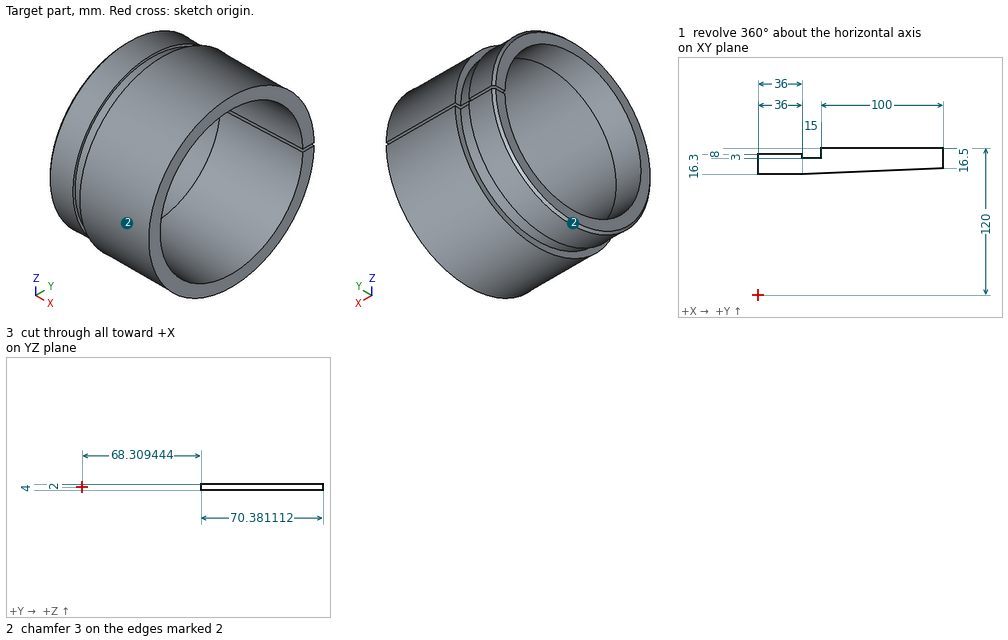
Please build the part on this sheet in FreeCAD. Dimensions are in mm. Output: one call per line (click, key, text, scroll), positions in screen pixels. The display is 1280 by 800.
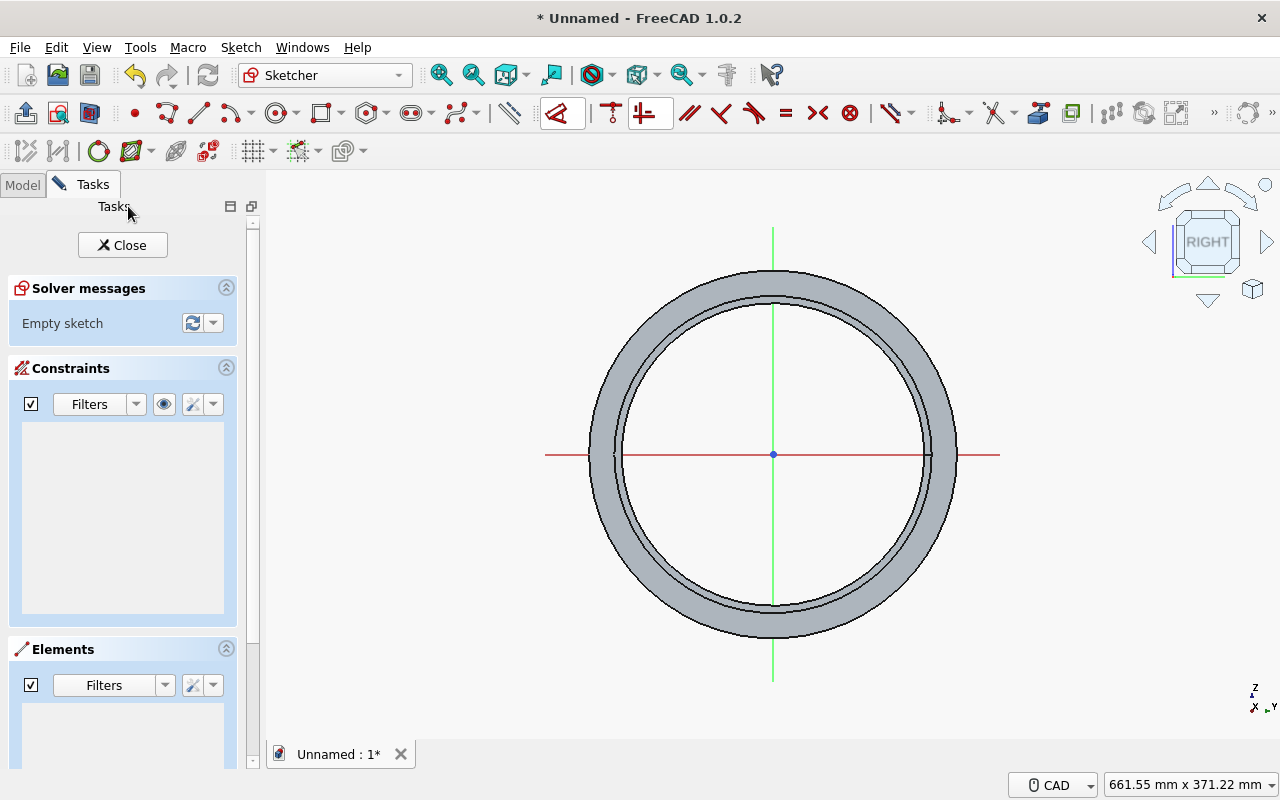
click(90, 114)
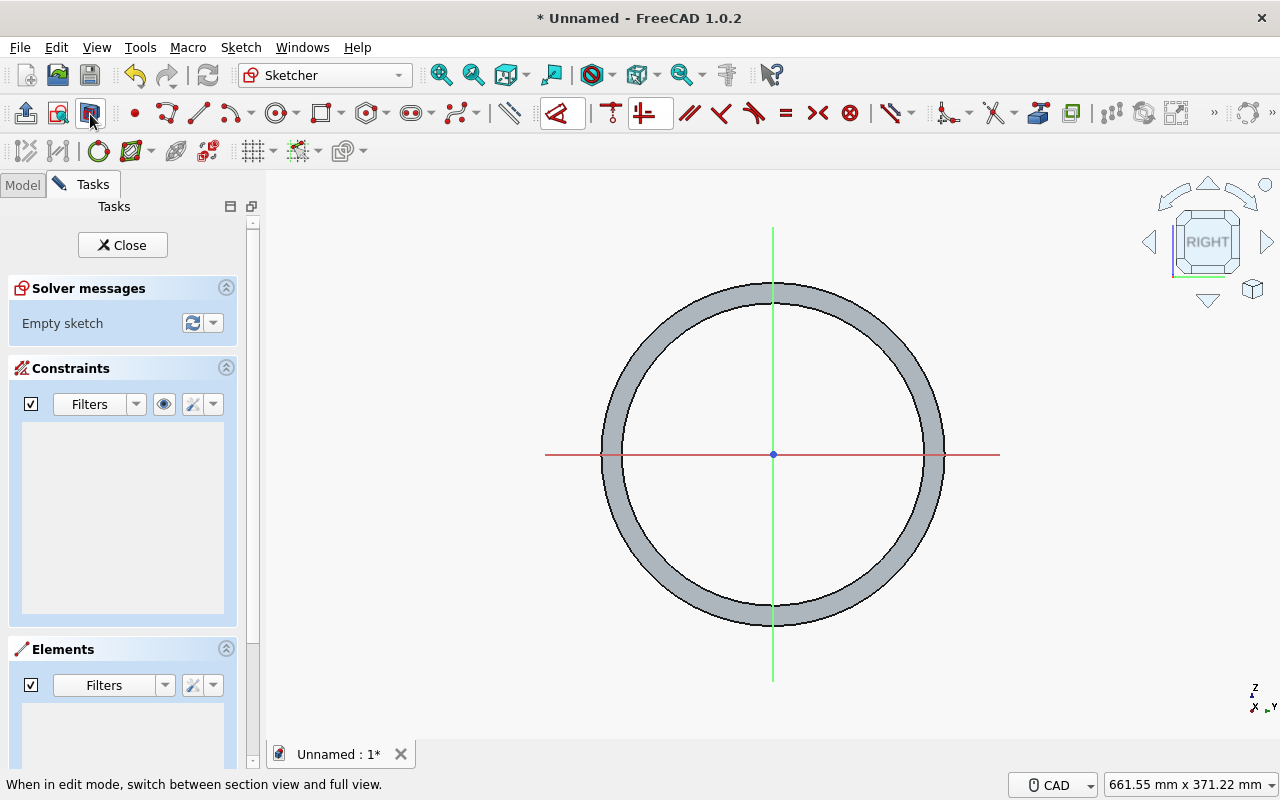
scroll(981, 454, up, 5)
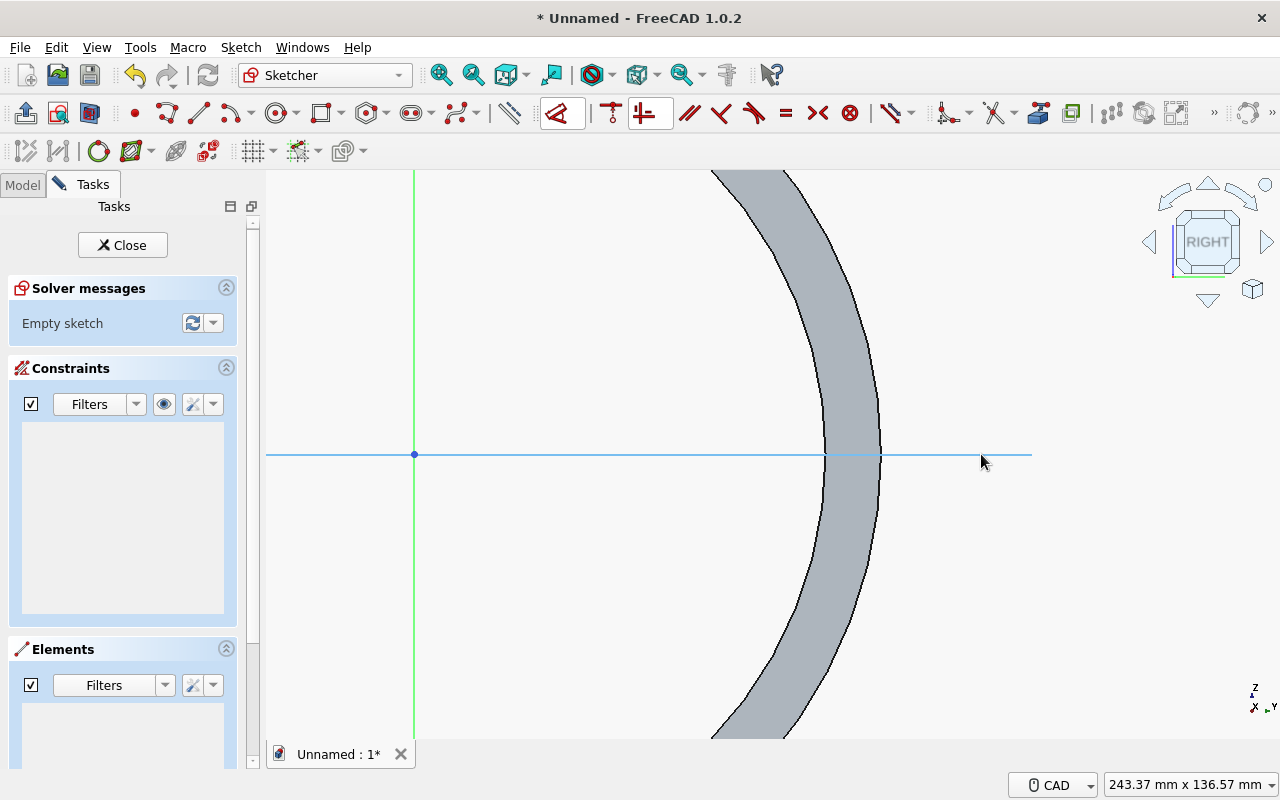
click(322, 114)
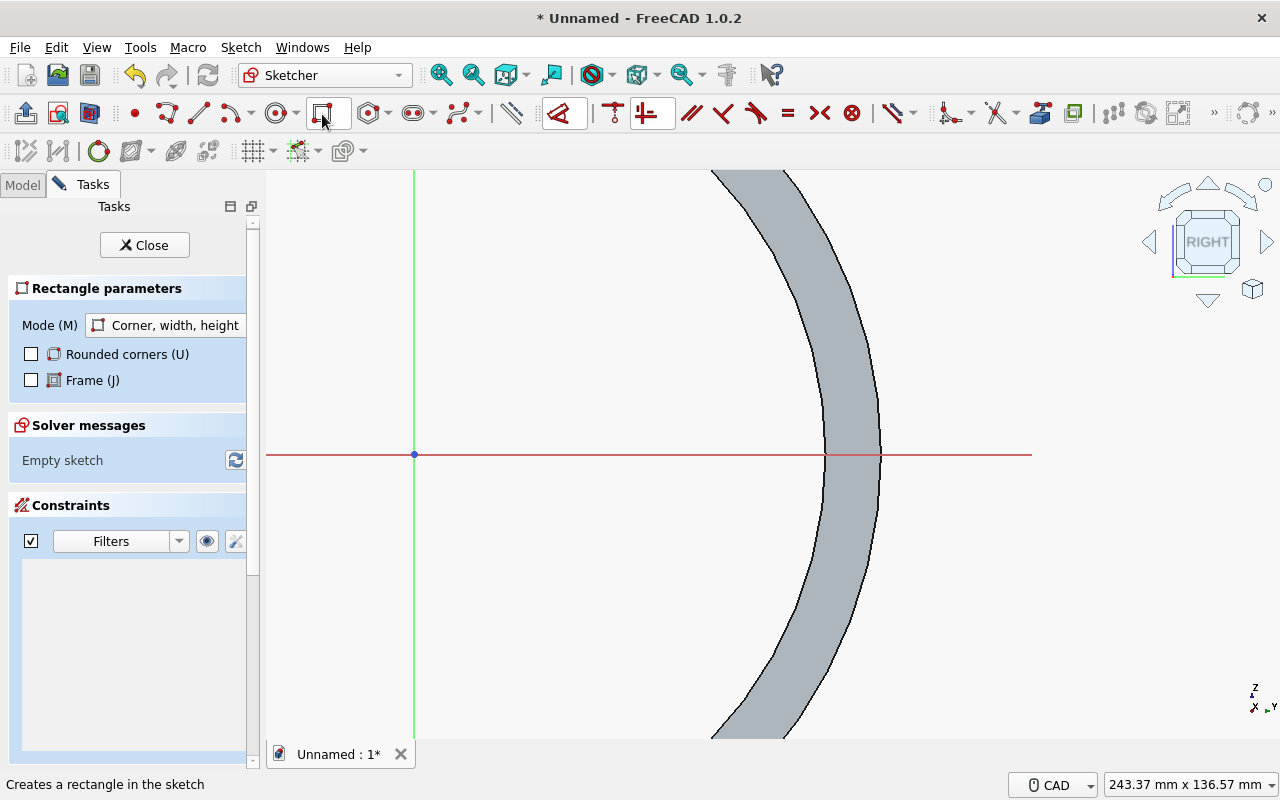
scroll(699, 446, up, 4)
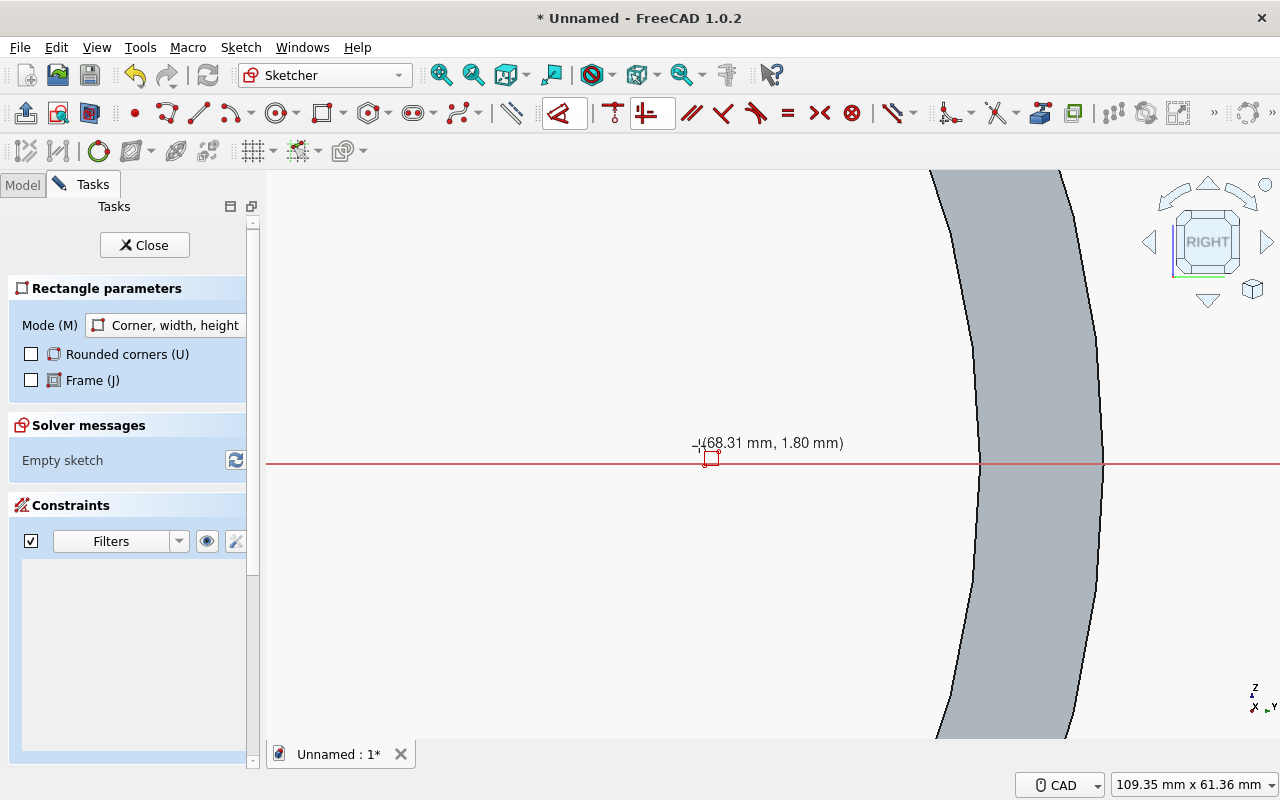
click(698, 446)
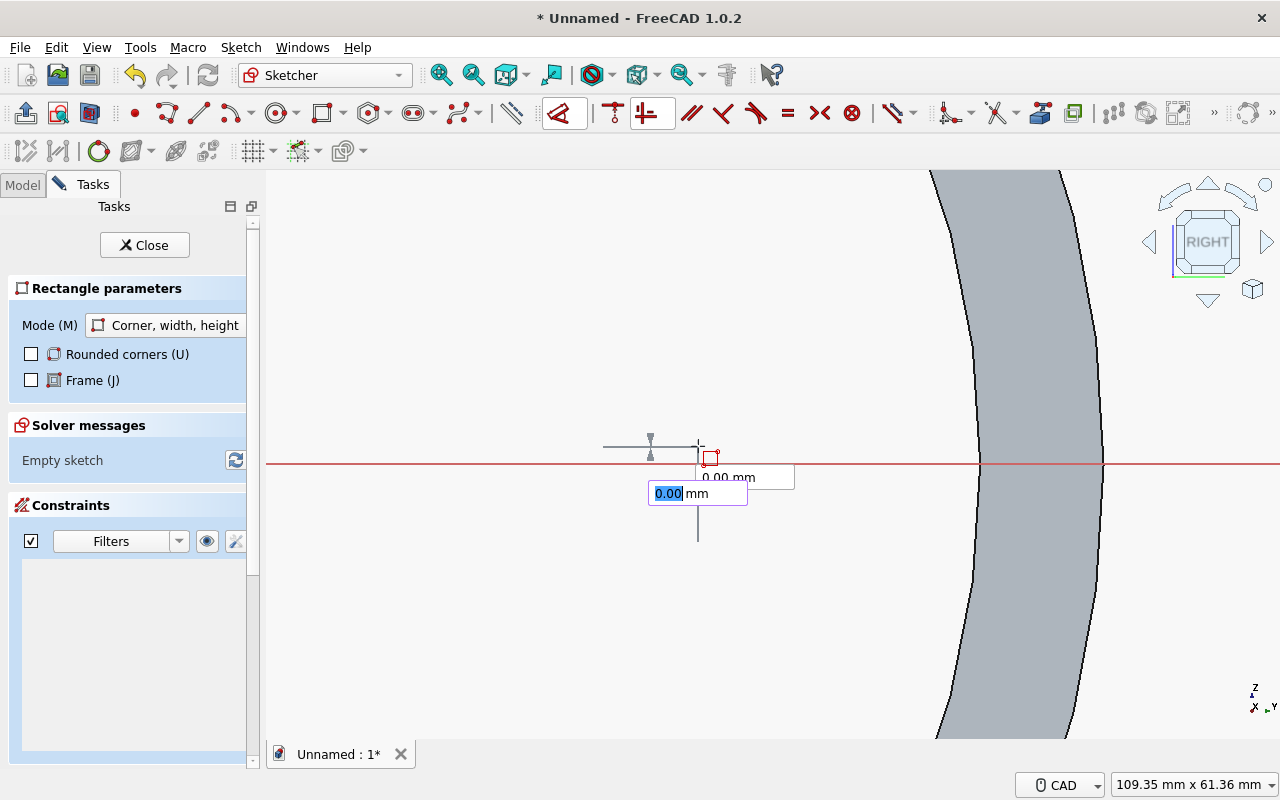
scroll(702, 446, down, 4)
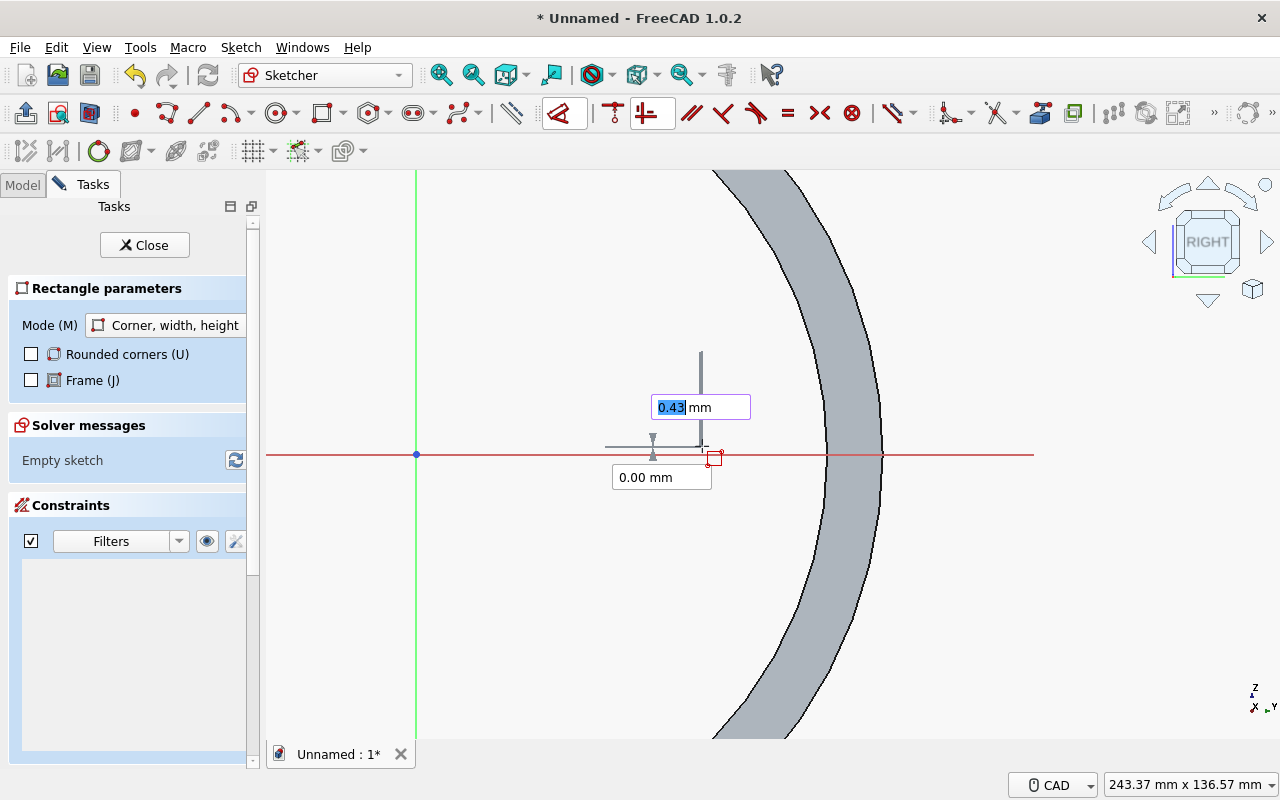
scroll(994, 463, up, 4)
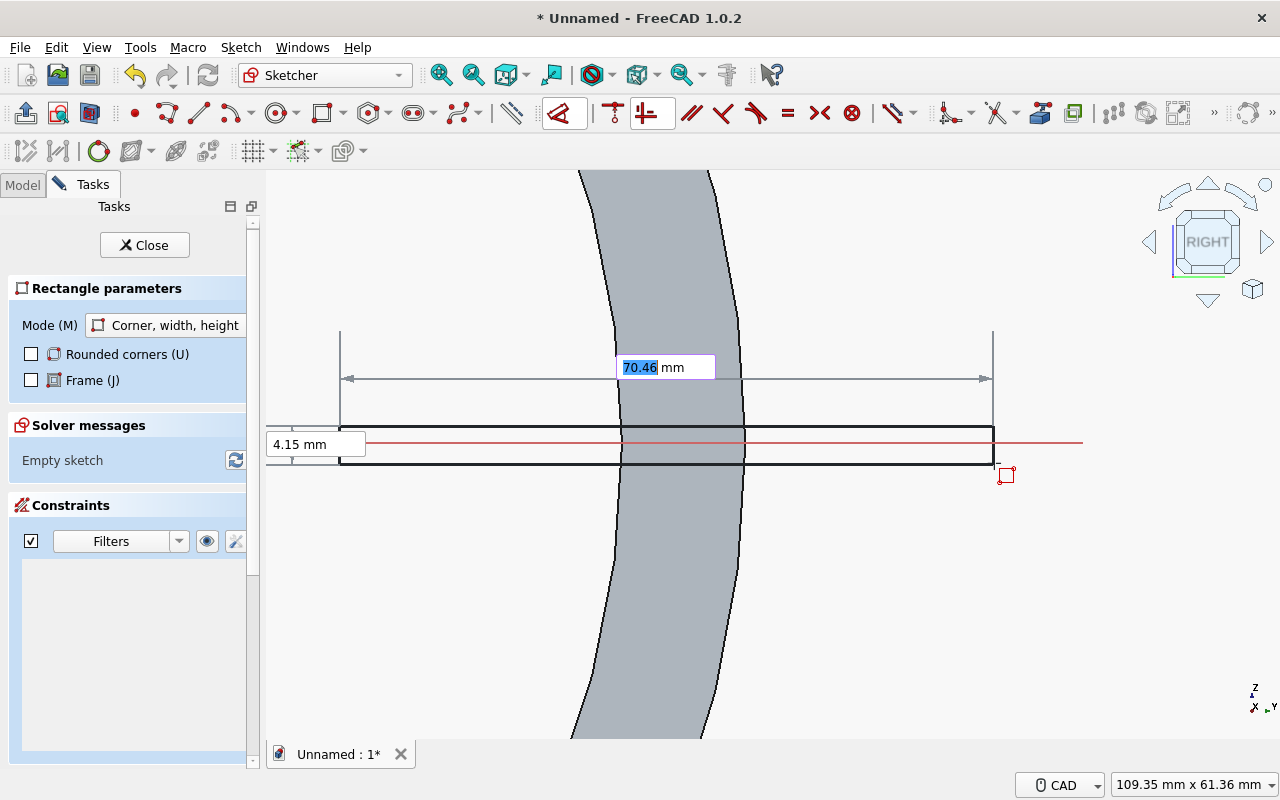
click(993, 462)
key(Escape)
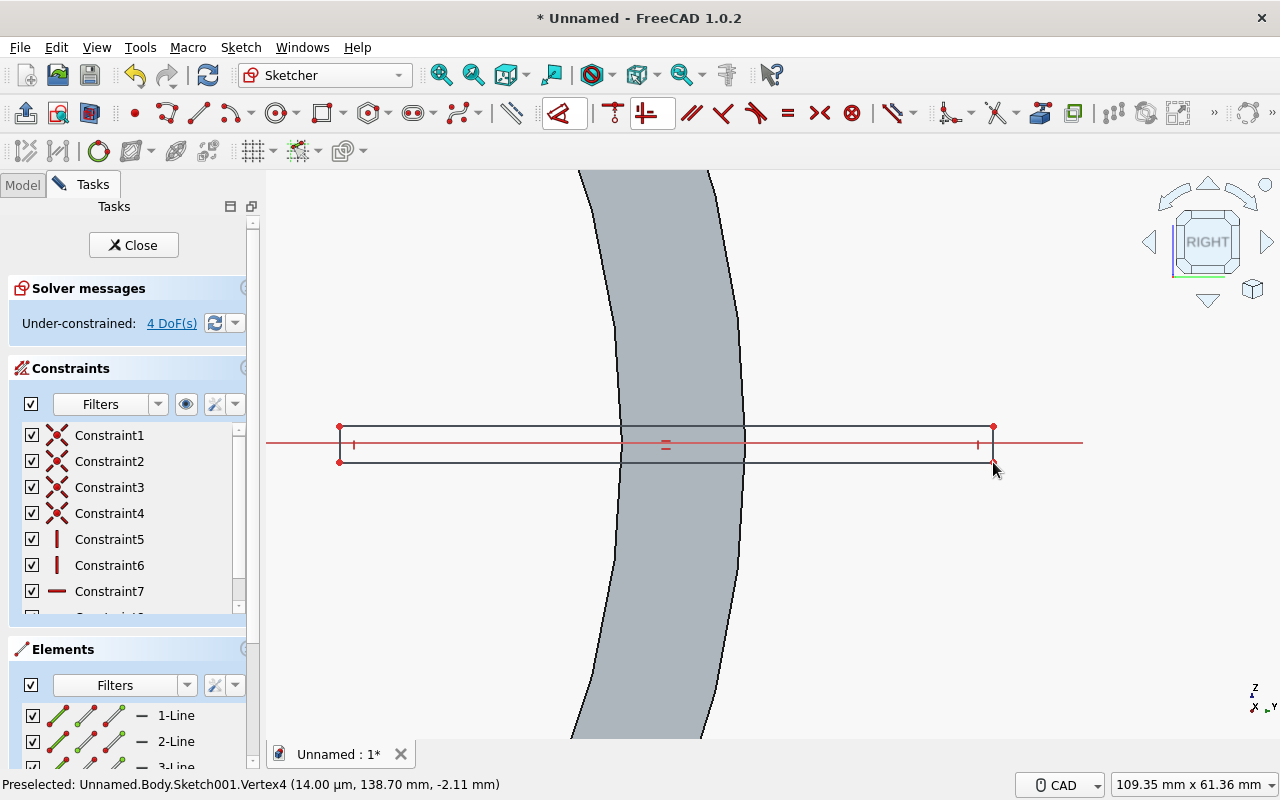
click(340, 441)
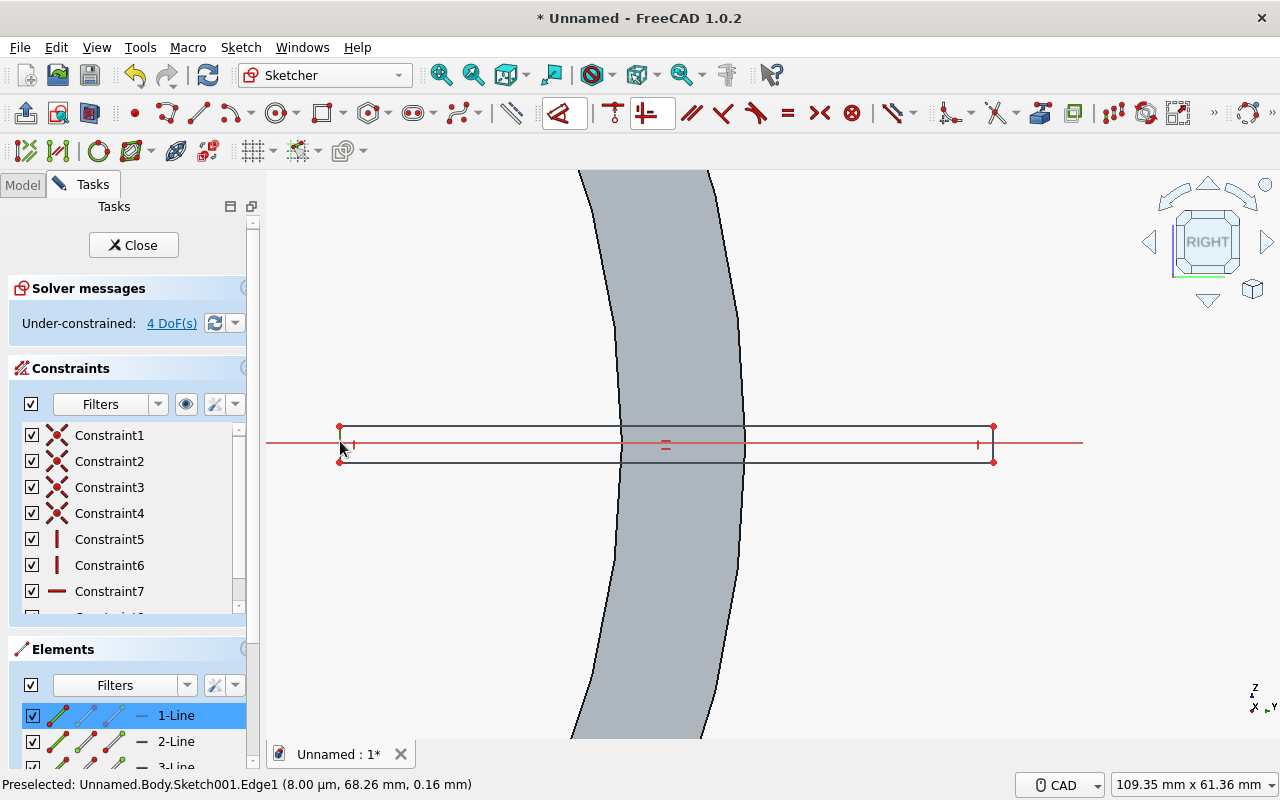
key(i)